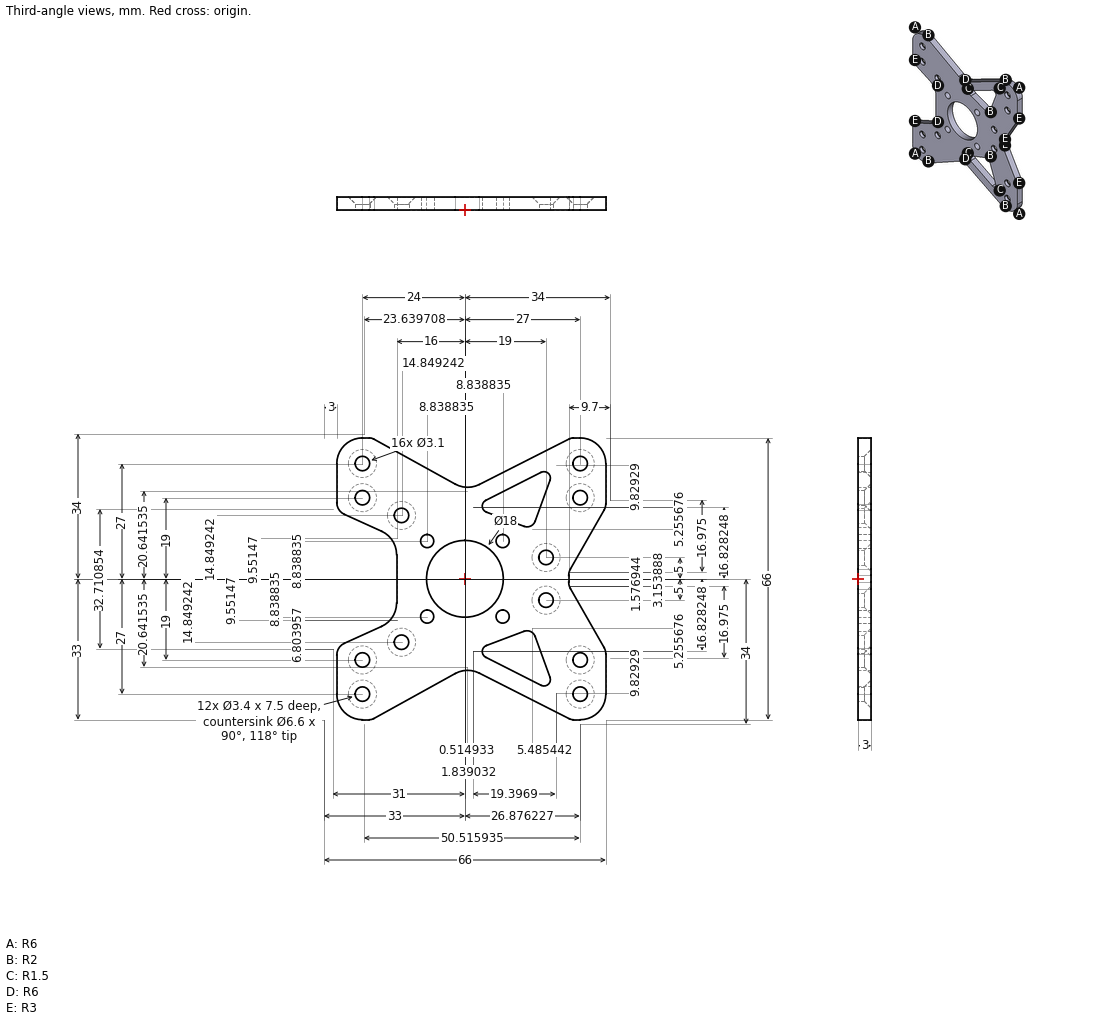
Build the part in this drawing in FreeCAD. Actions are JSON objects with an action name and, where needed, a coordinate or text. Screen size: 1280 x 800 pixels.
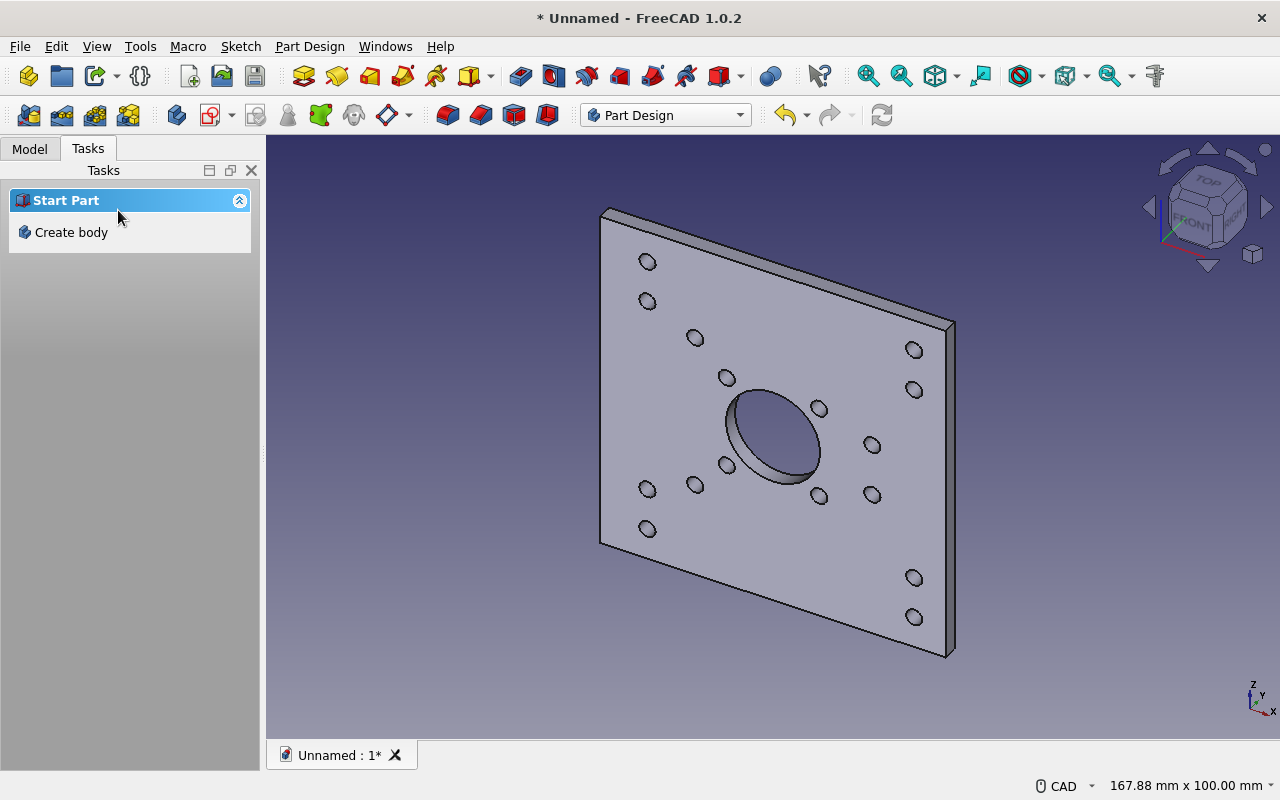
{"action": "key", "text": "4"}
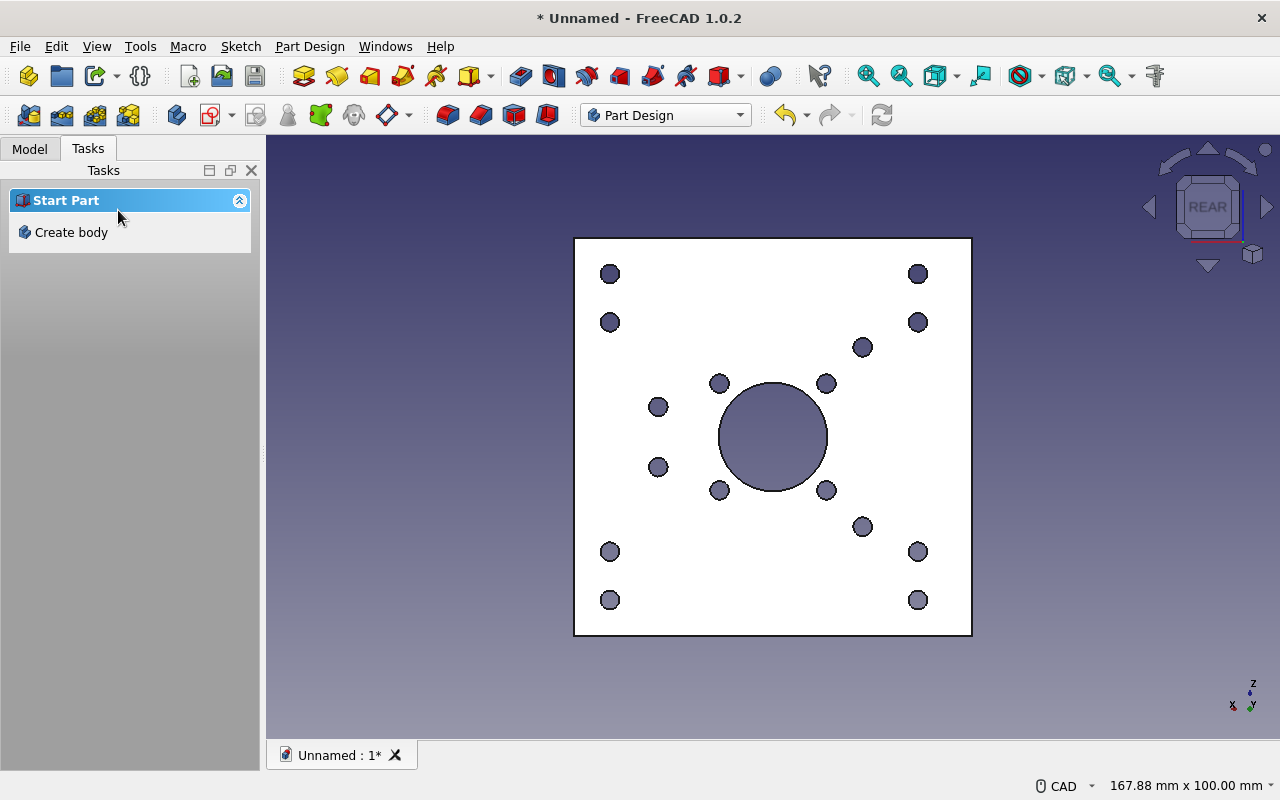
{"action": "left_click", "coordinate": [887, 436]}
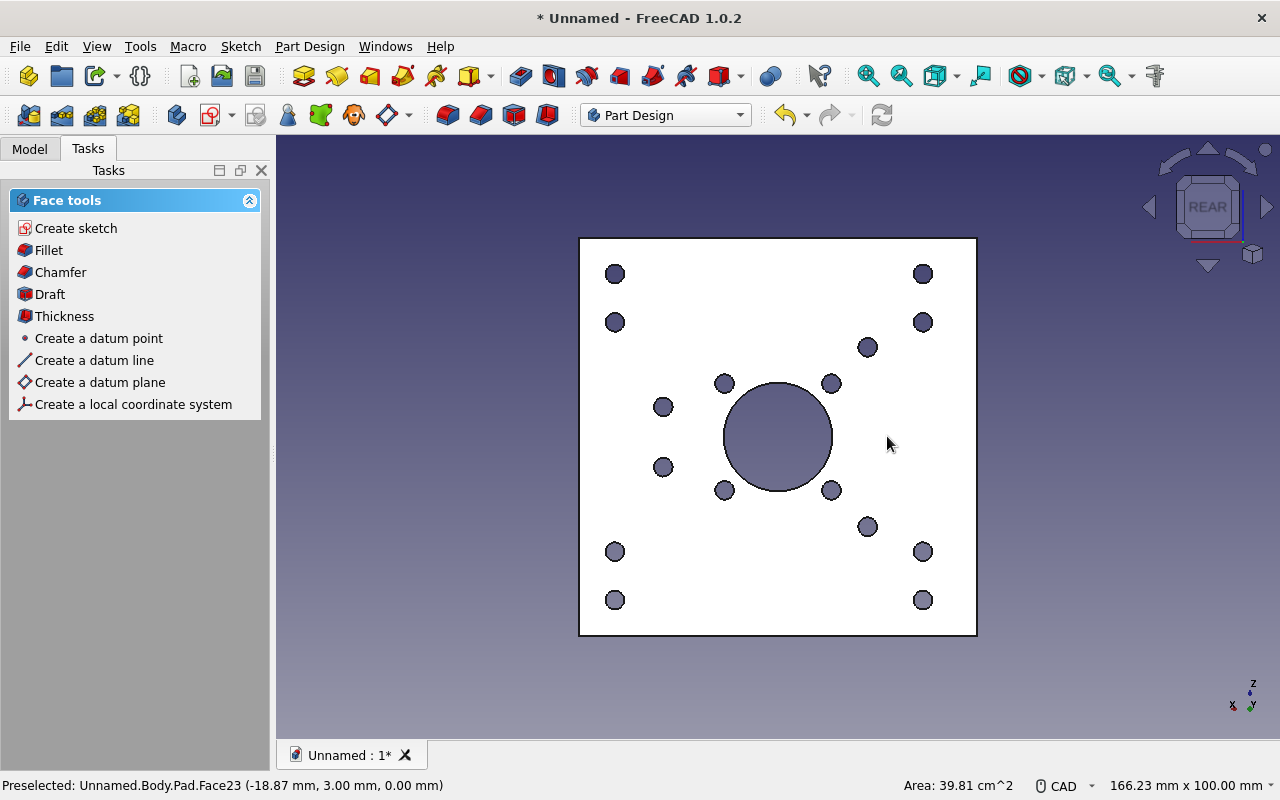
{"action": "left_click", "coordinate": [210, 116]}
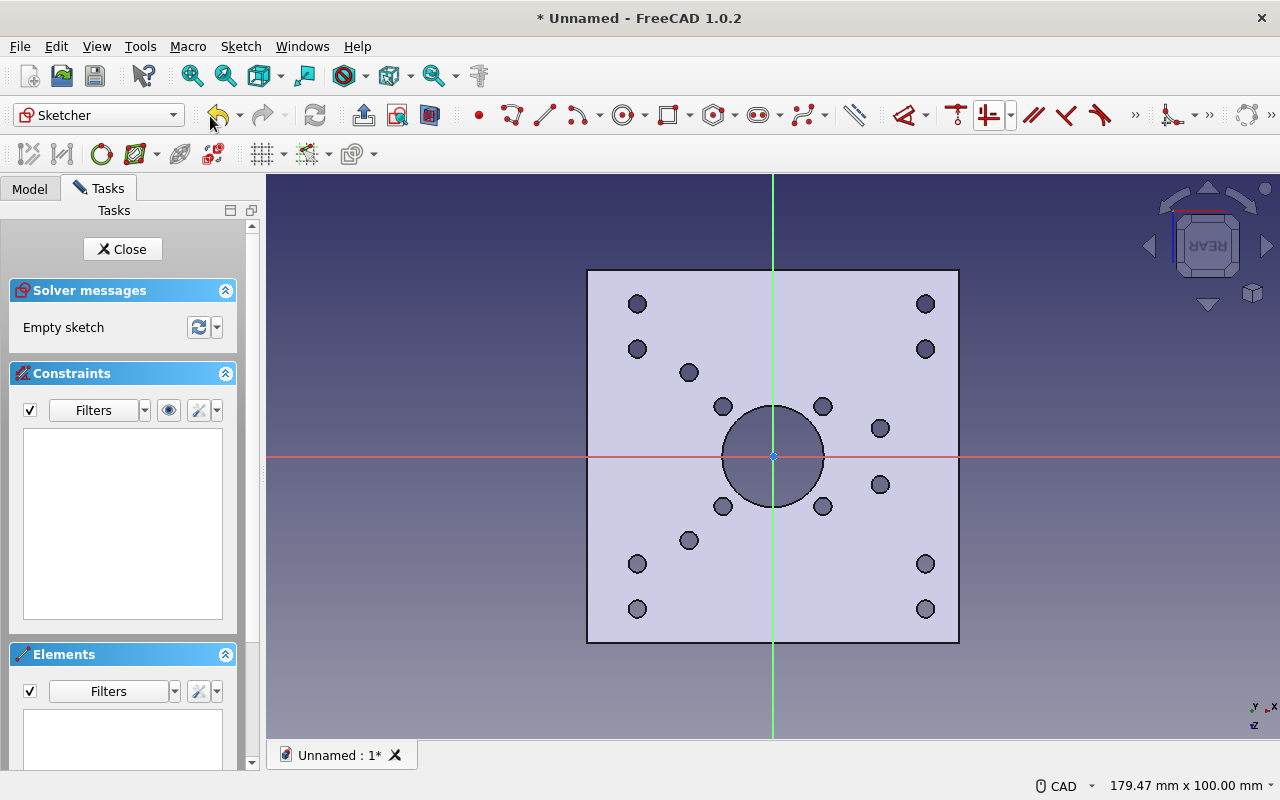
{"action": "left_click", "coordinate": [622, 116]}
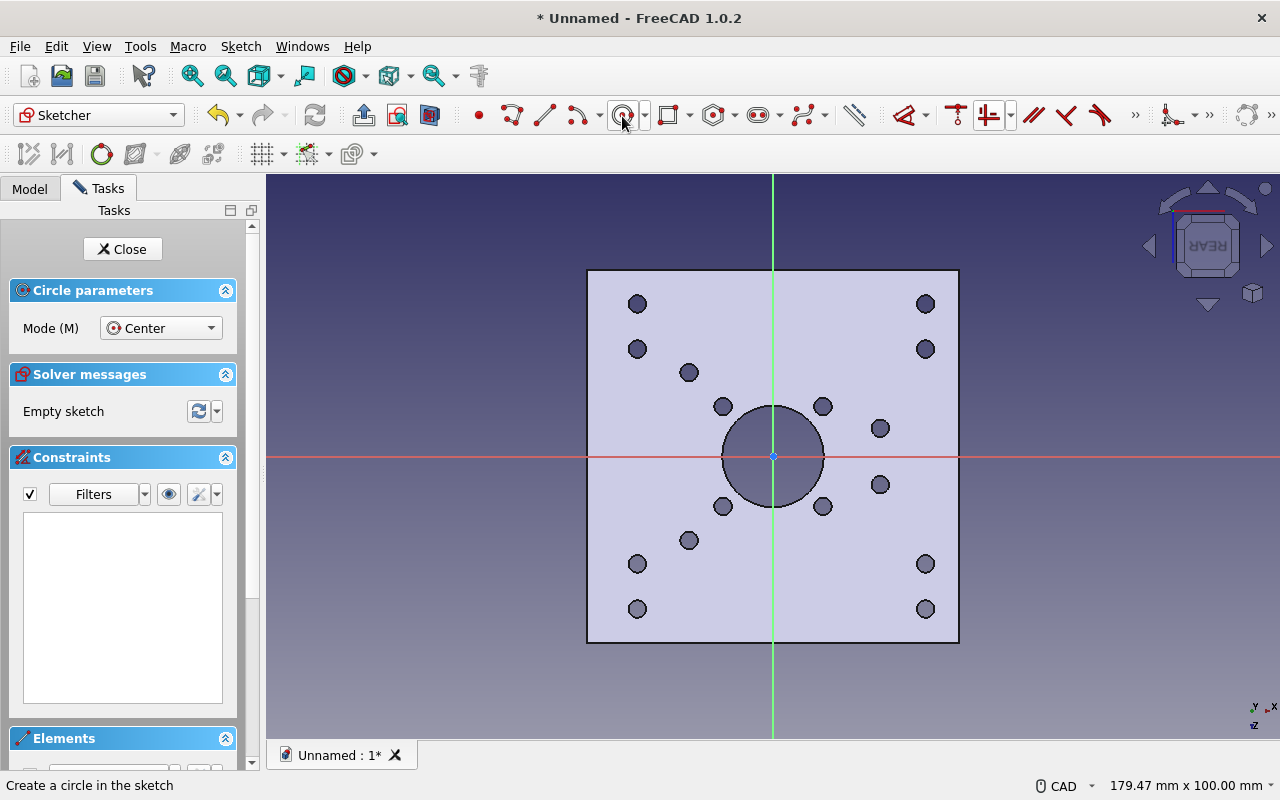
{"action": "scroll", "coordinate": [637, 304], "scroll_direction": "up", "scroll_amount": 5}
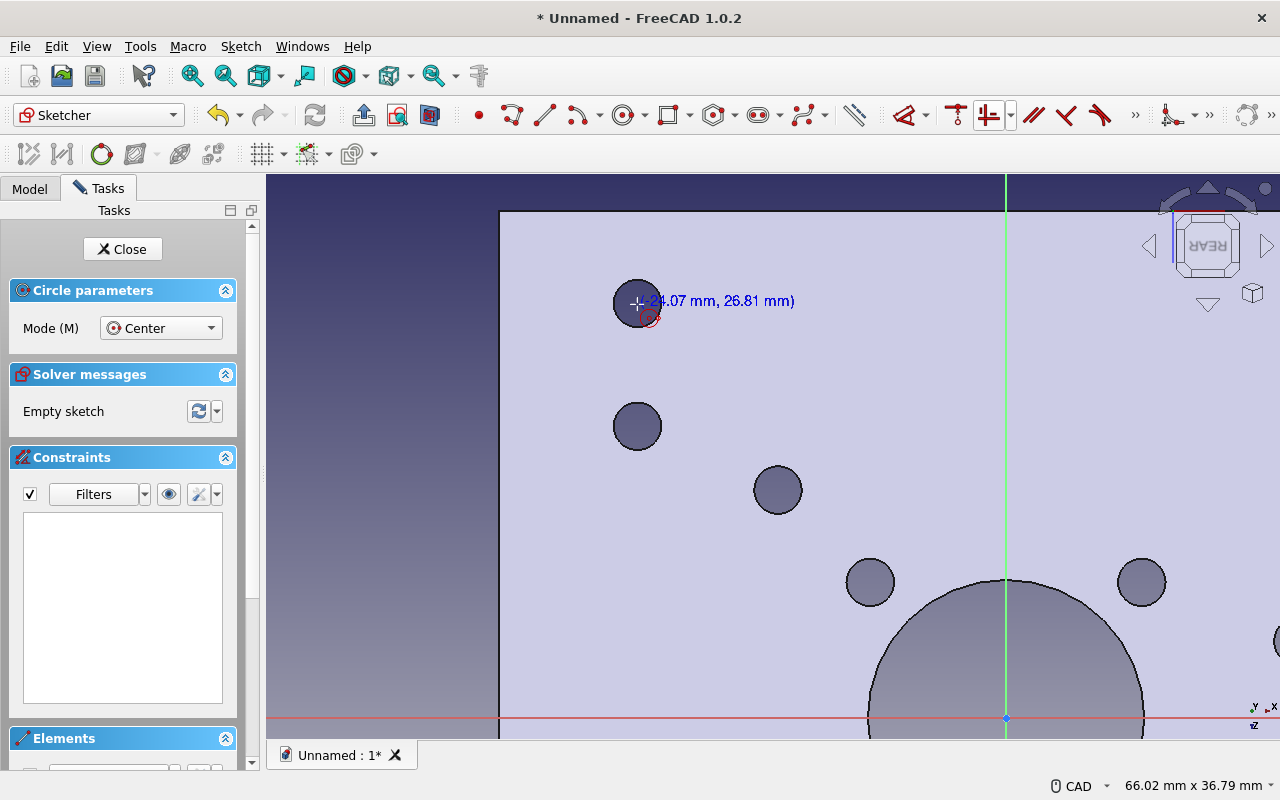
{"action": "left_click", "coordinate": [637, 303]}
{"action": "mouse_move", "coordinate": [656, 285]}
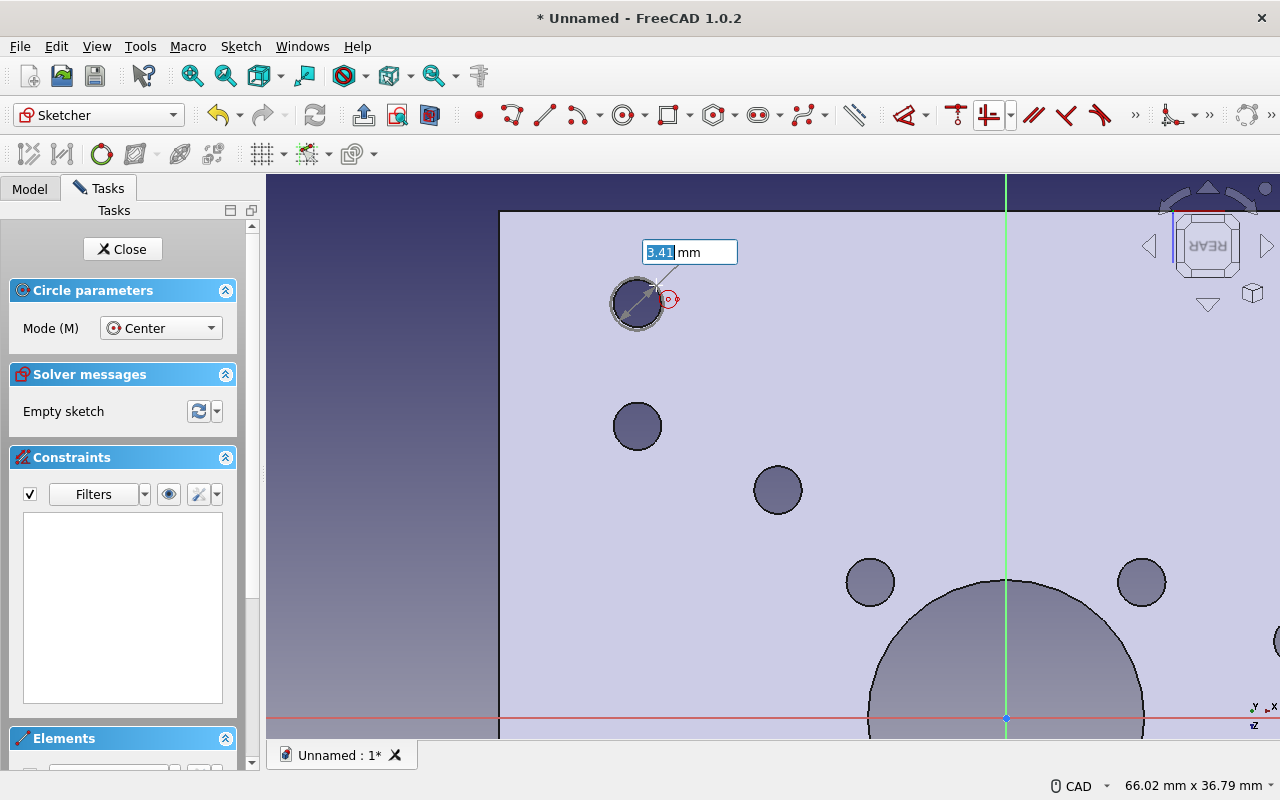
{"action": "type", "text": "3.4"}
{"action": "key", "text": "Return"}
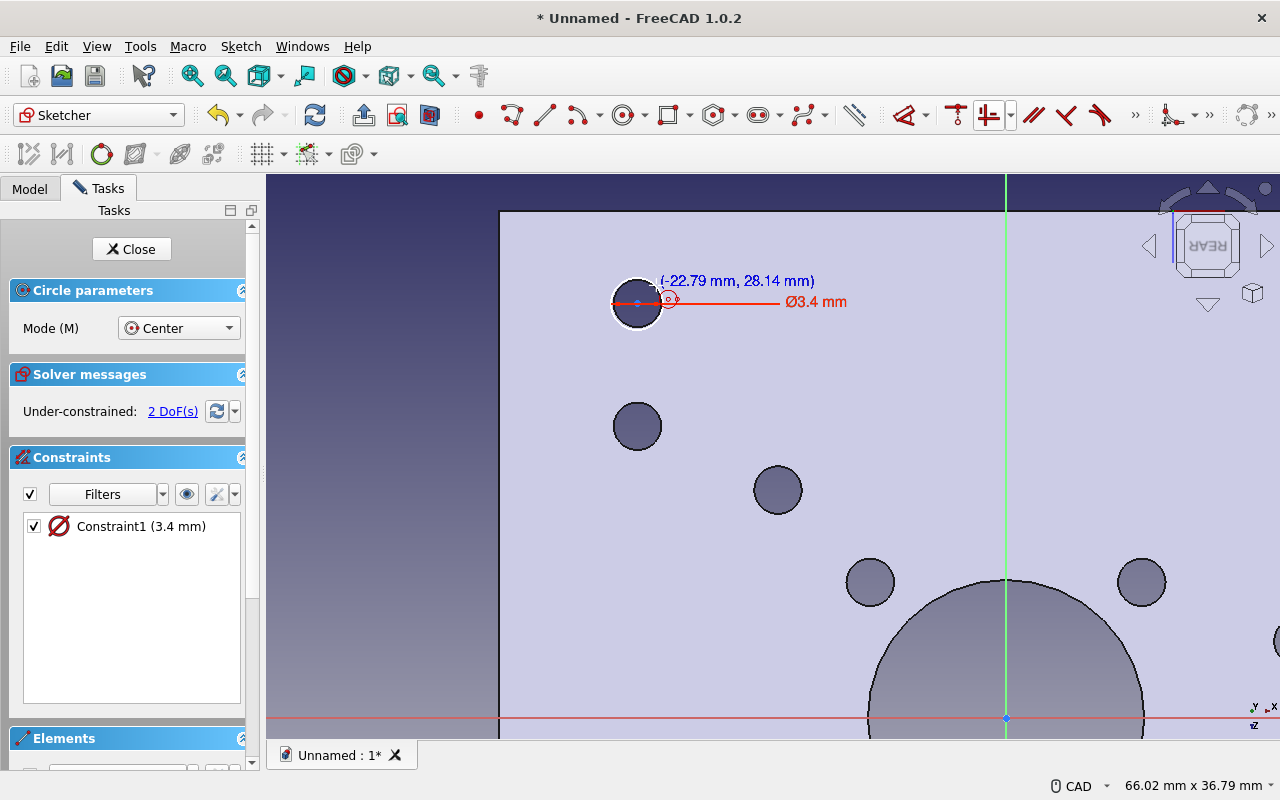
{"action": "left_click", "coordinate": [637, 426]}
{"action": "mouse_move", "coordinate": [656, 408]}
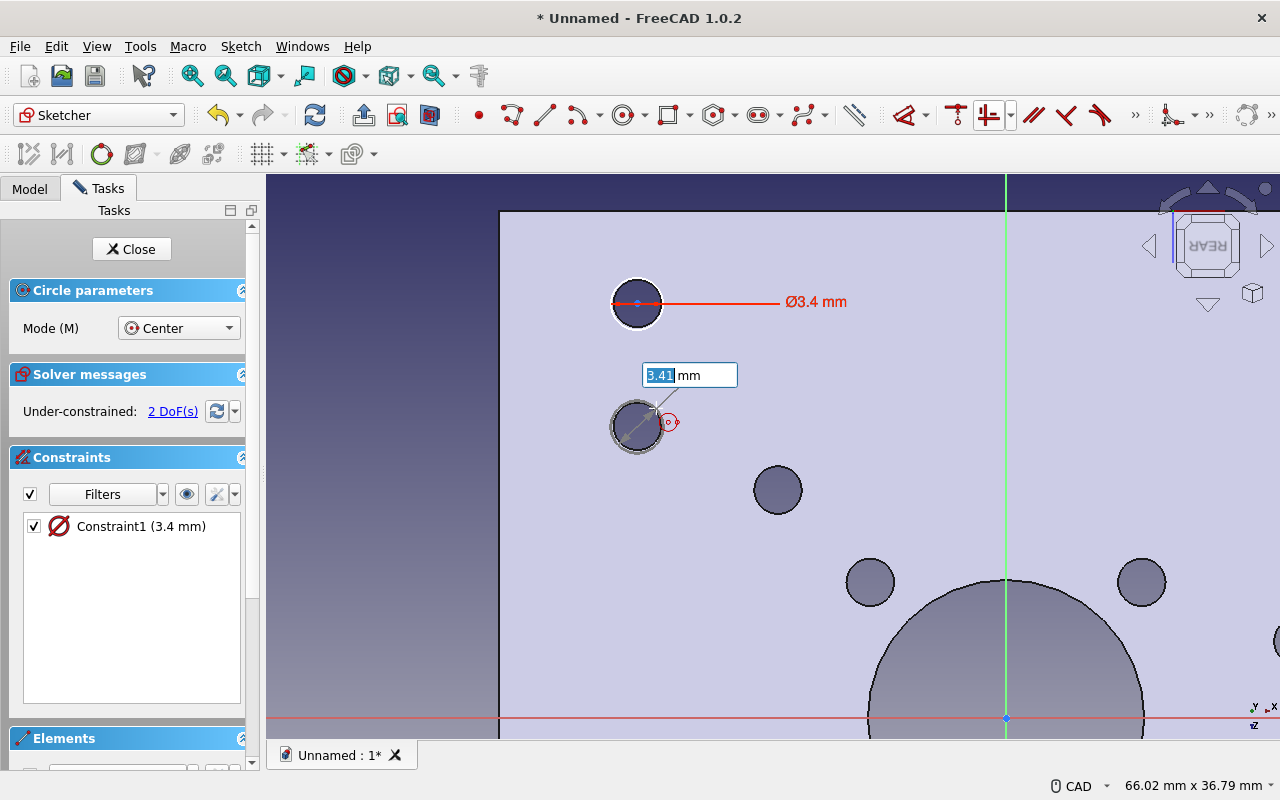
{"action": "type", "text": "3.4"}
{"action": "key", "text": "Return"}